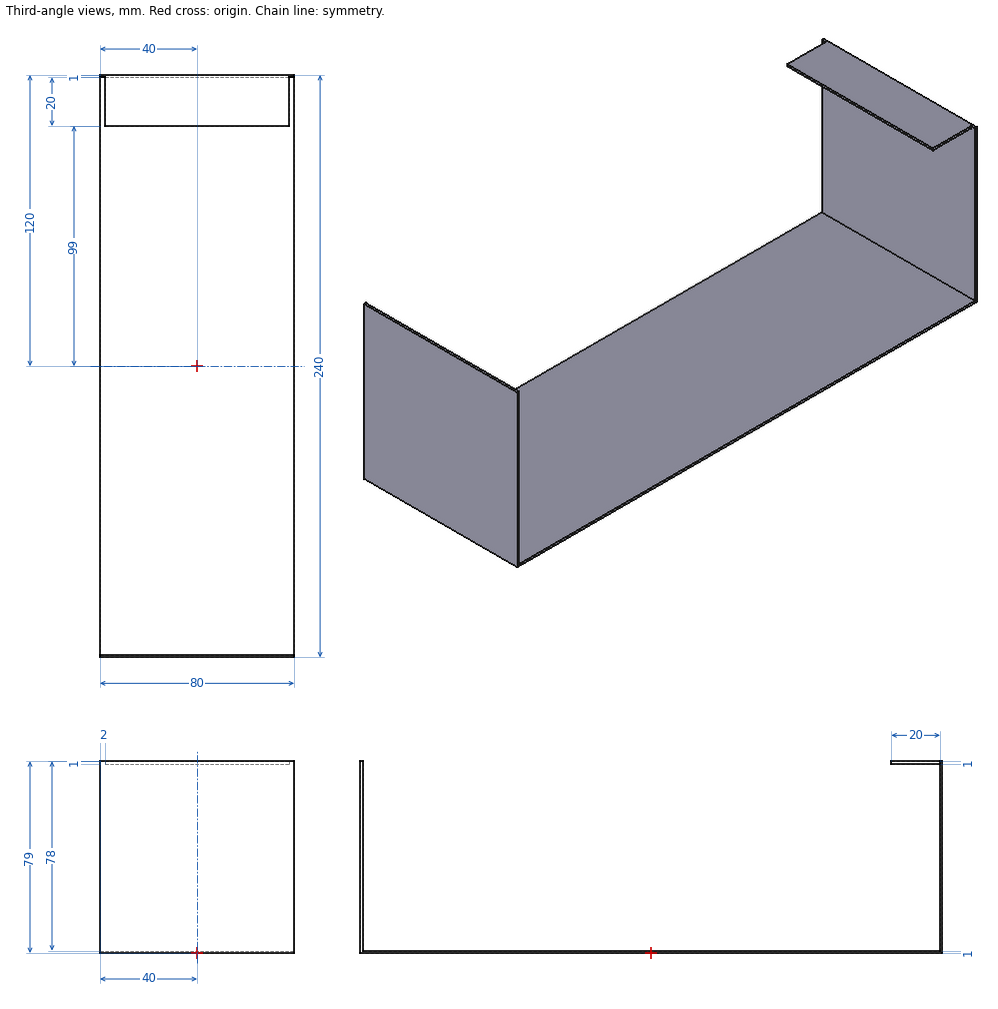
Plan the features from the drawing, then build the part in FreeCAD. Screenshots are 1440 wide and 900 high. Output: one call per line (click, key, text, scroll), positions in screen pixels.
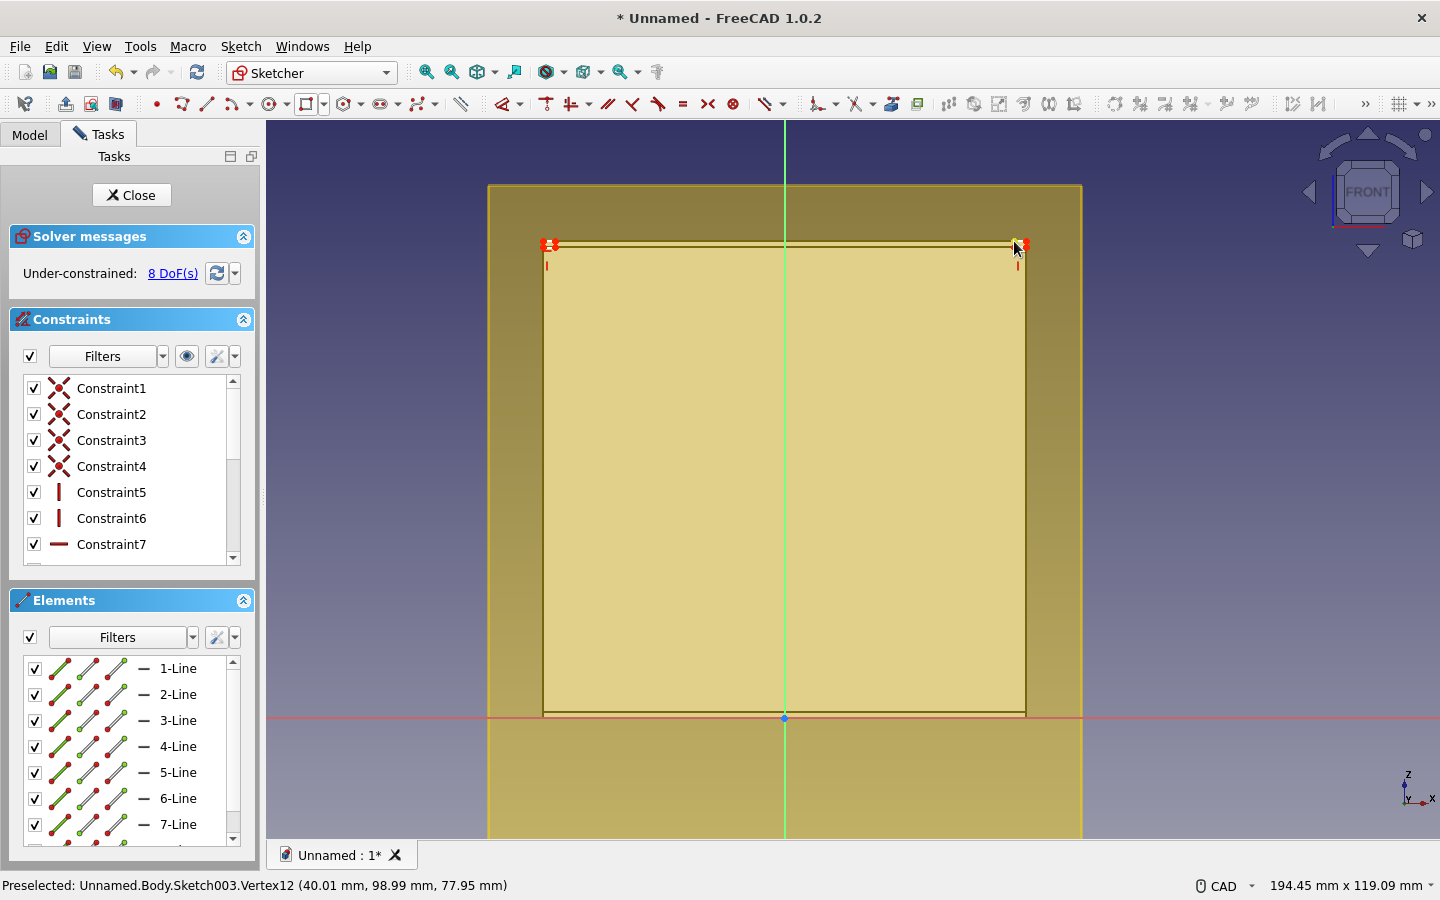
scroll(556, 241, up, 4)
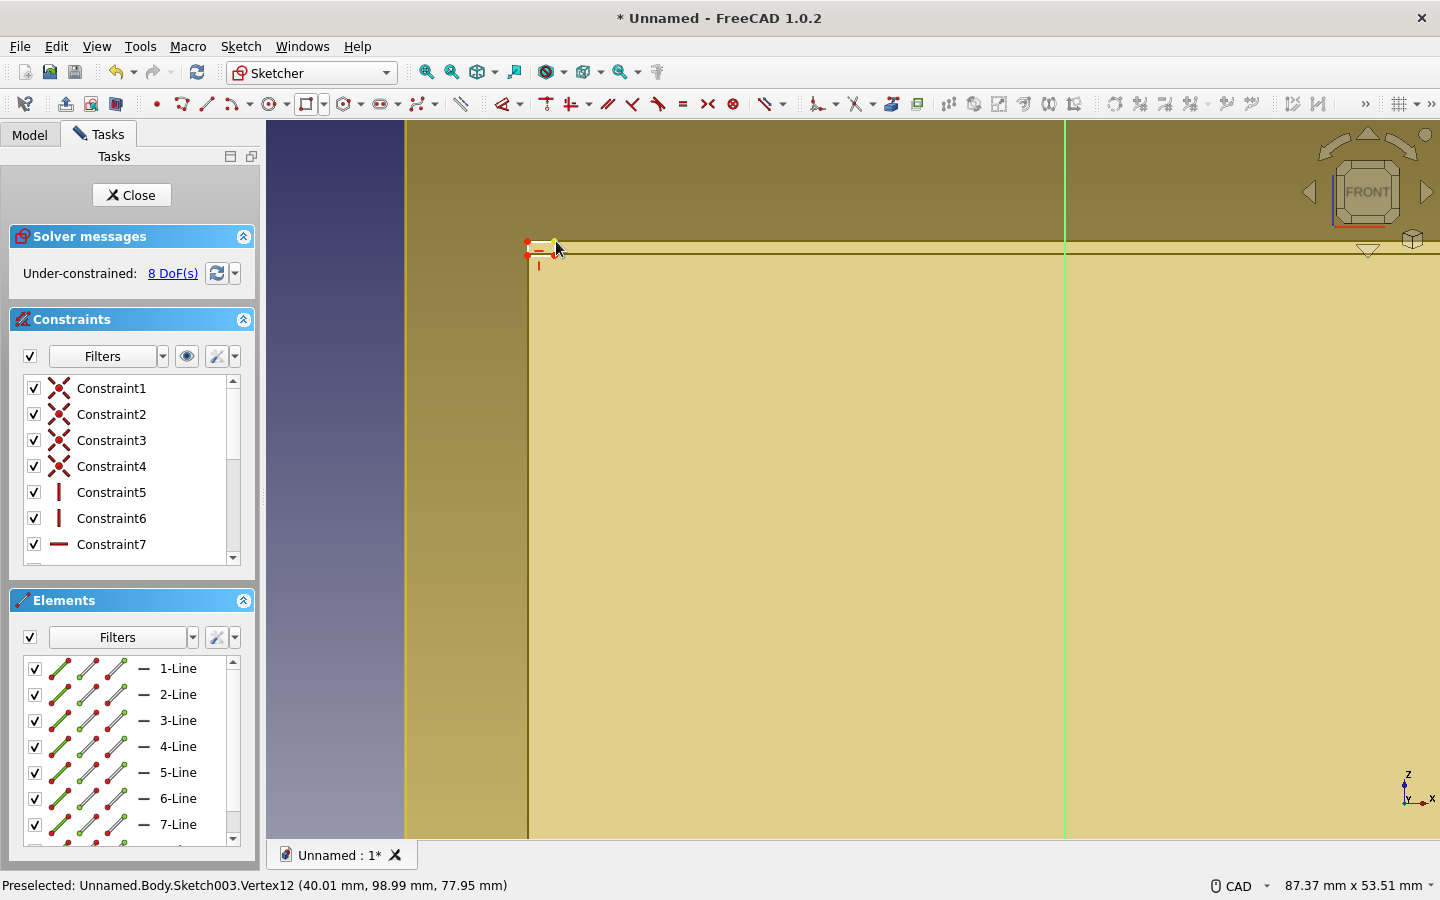
click(555, 242)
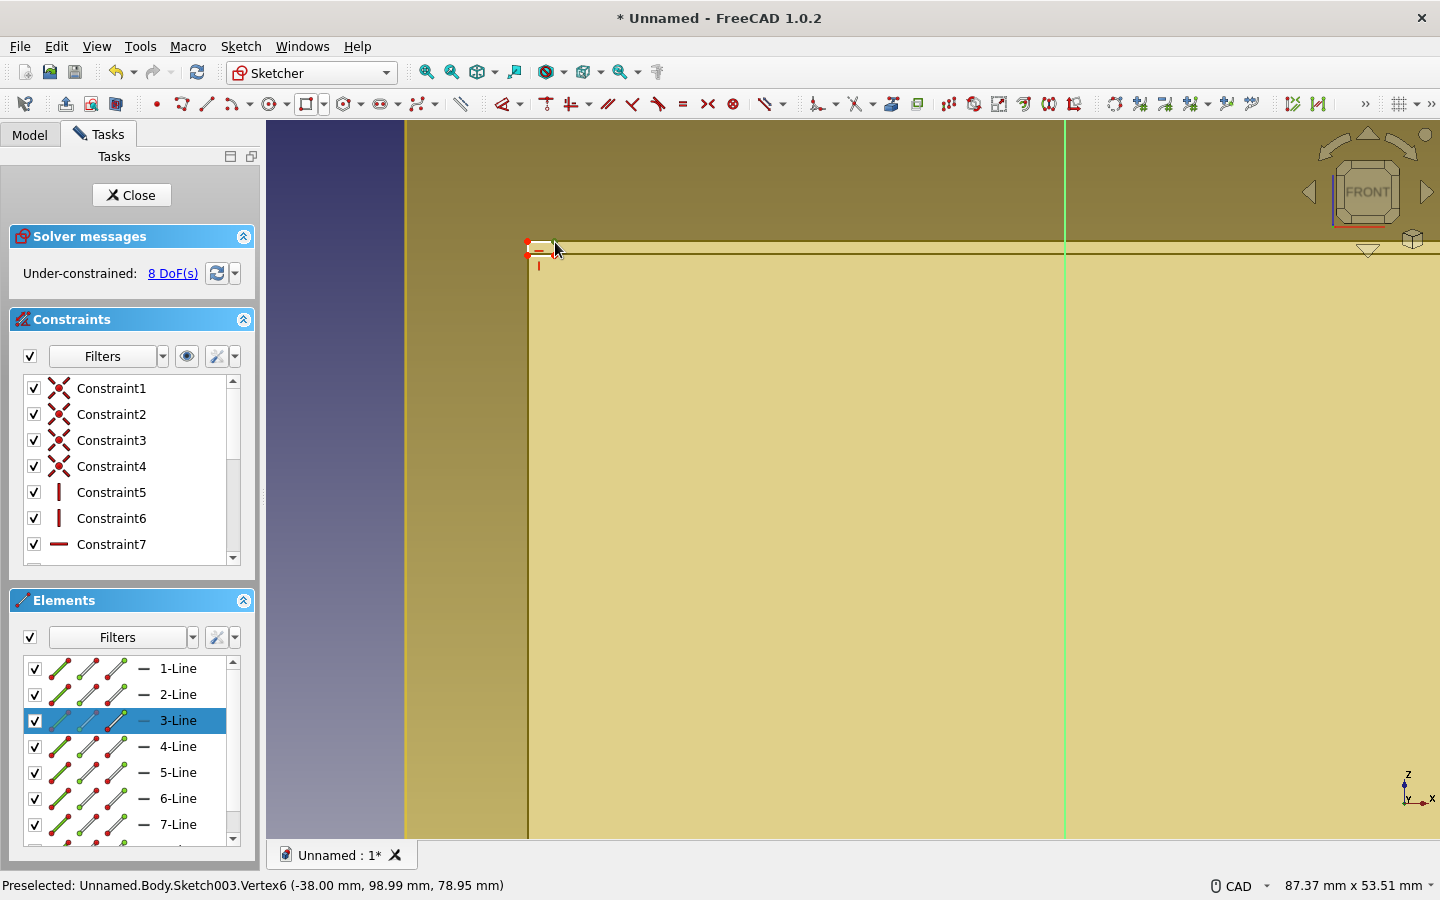
scroll(555, 241, down, 4)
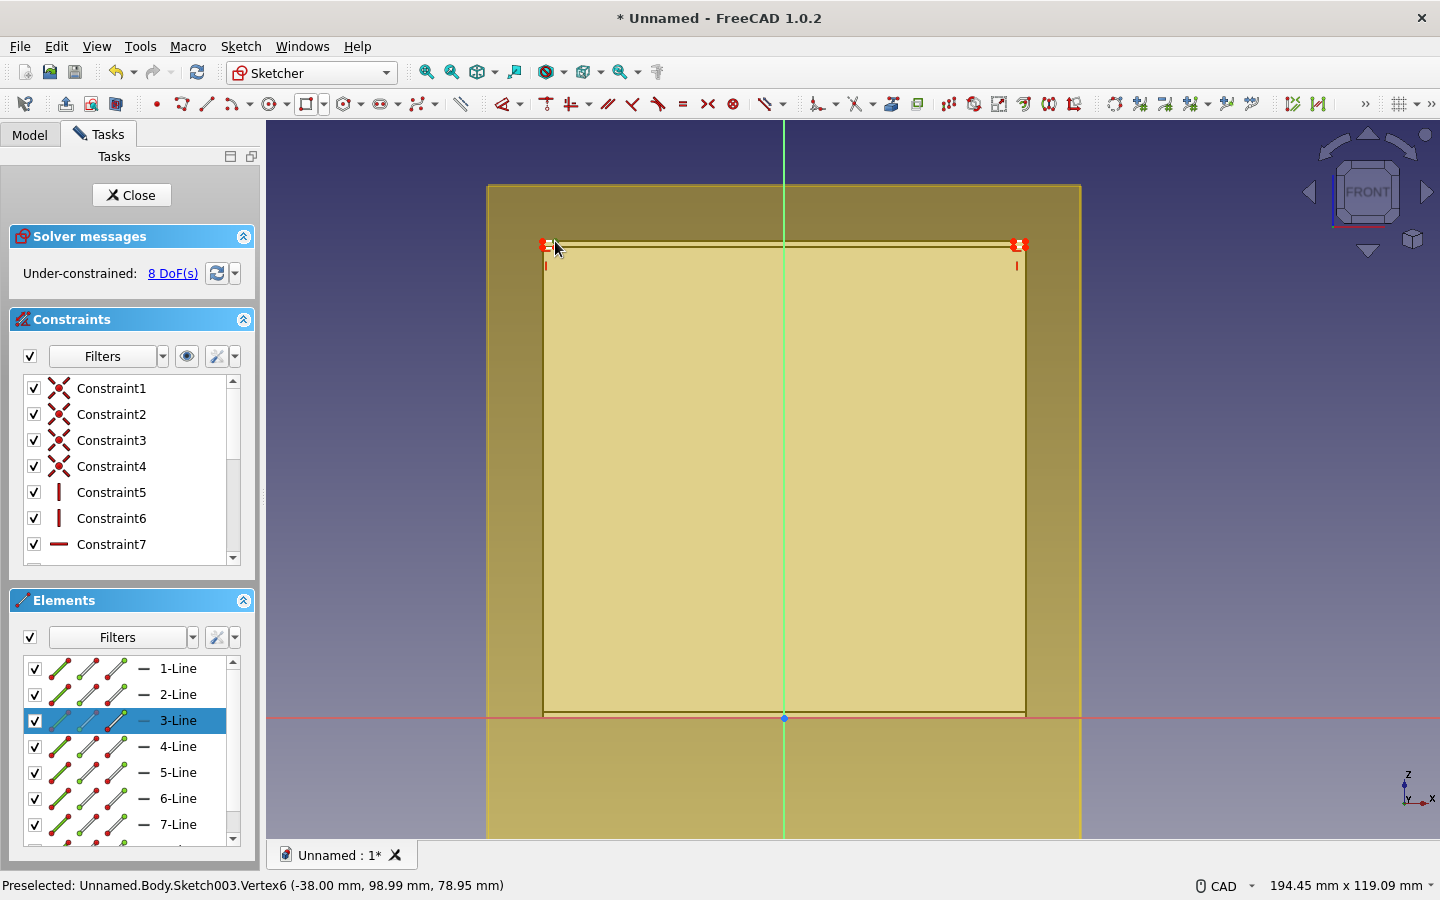
scroll(1014, 241, up, 4)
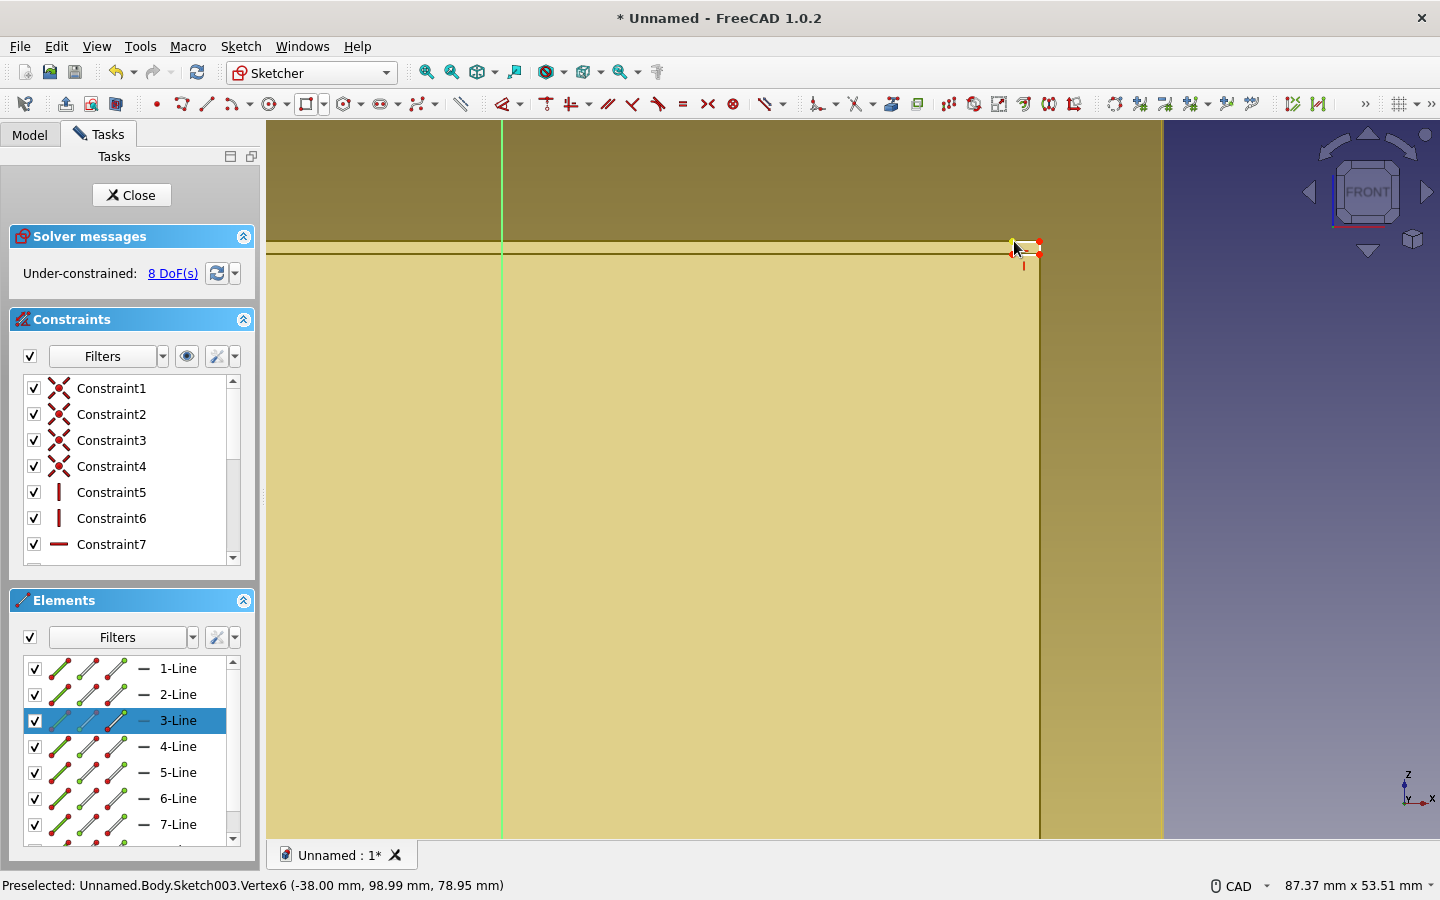
click(1013, 242)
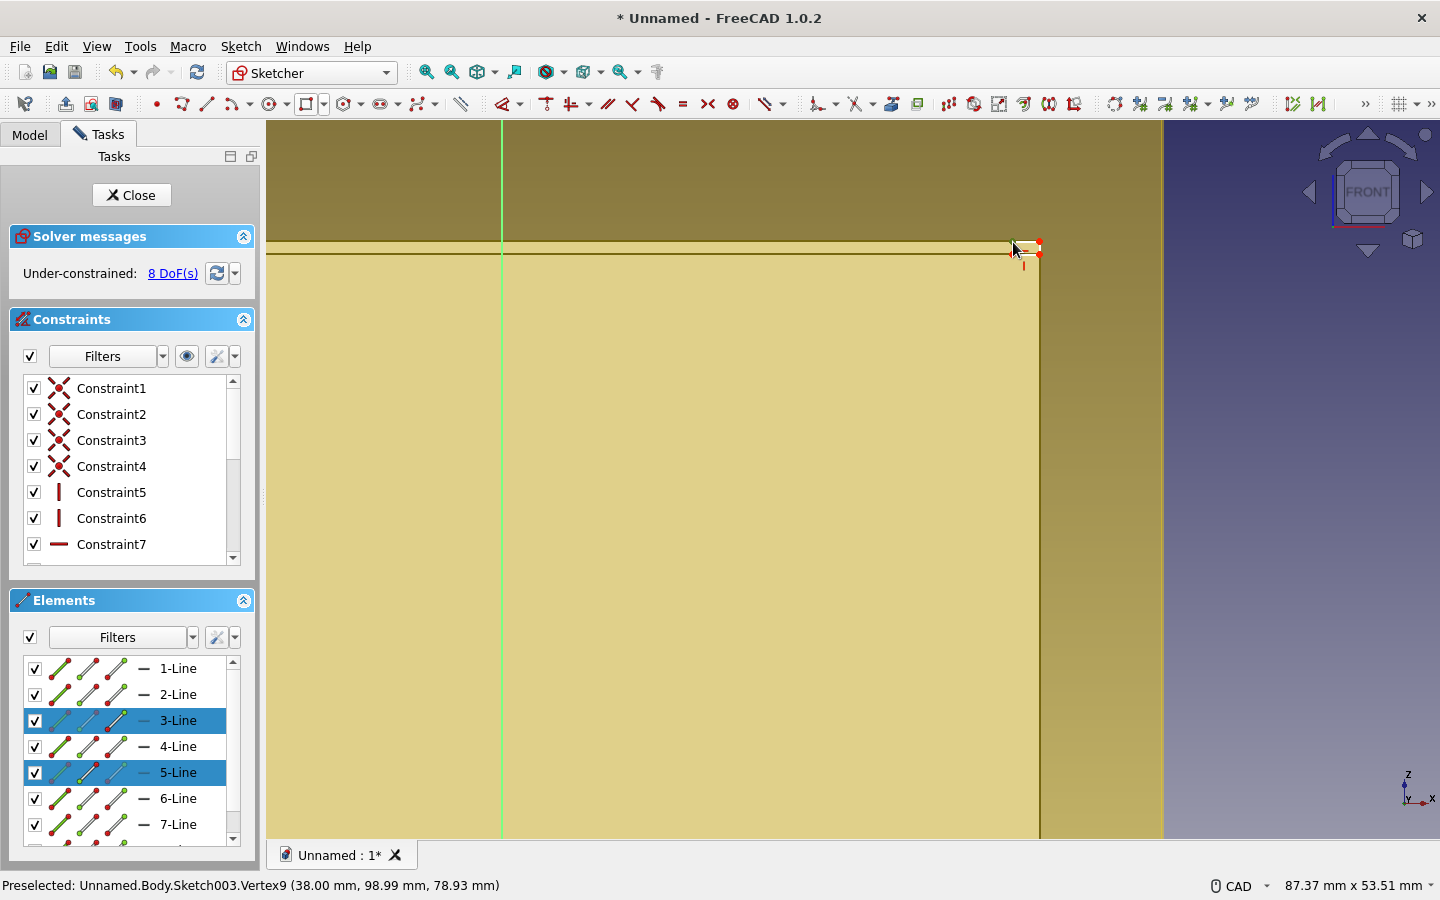
click(502, 764)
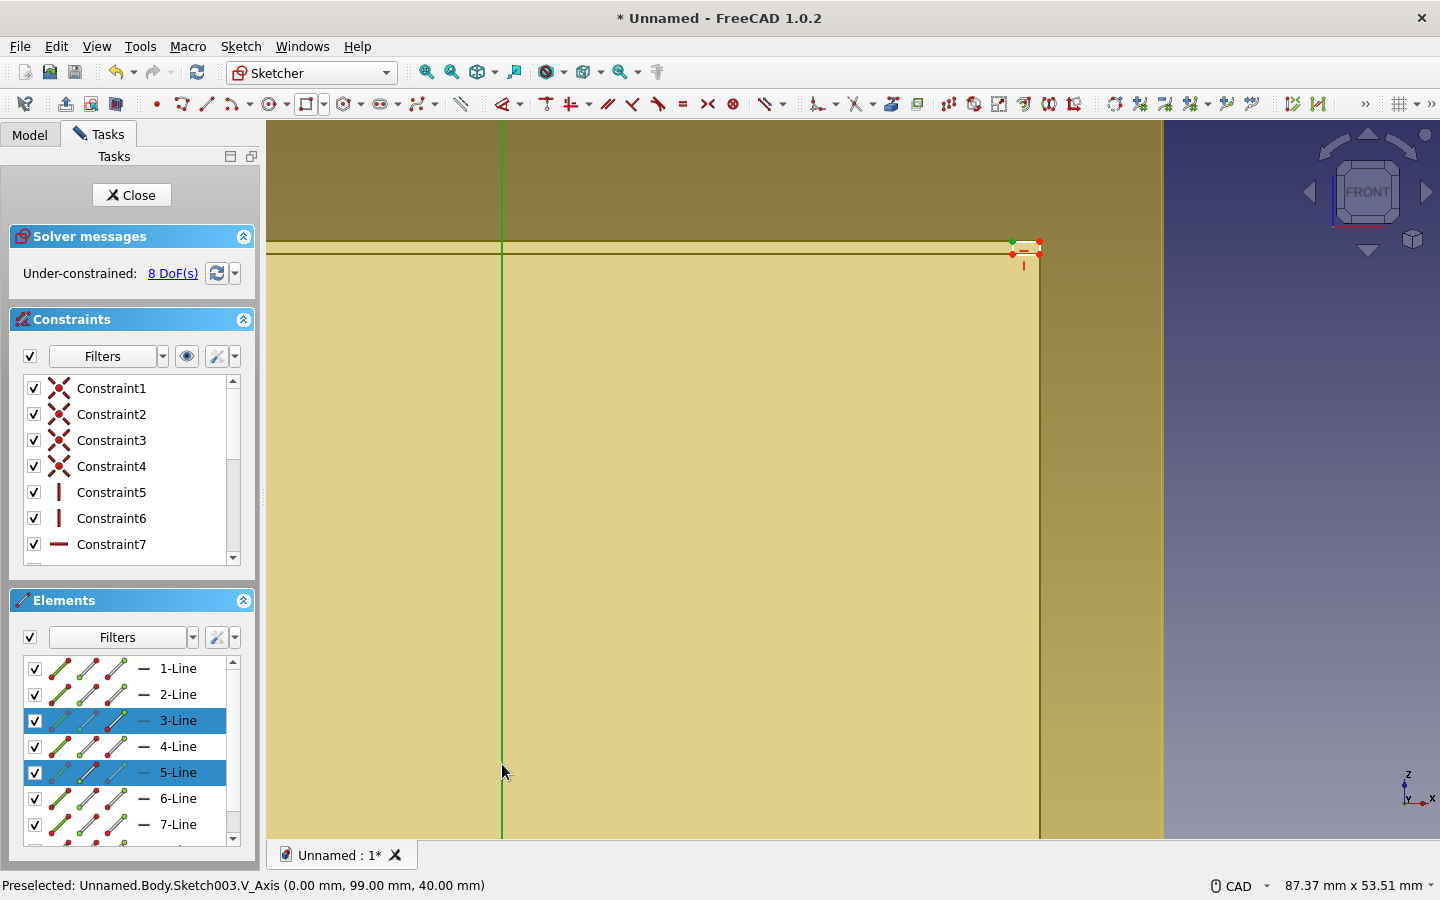
click(708, 104)